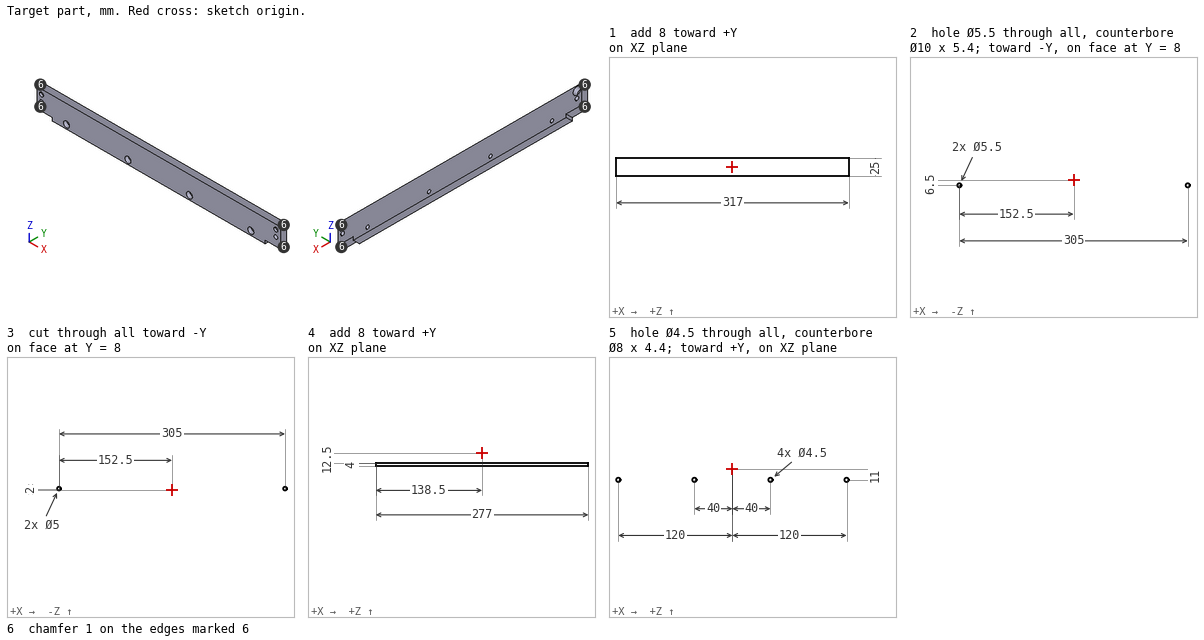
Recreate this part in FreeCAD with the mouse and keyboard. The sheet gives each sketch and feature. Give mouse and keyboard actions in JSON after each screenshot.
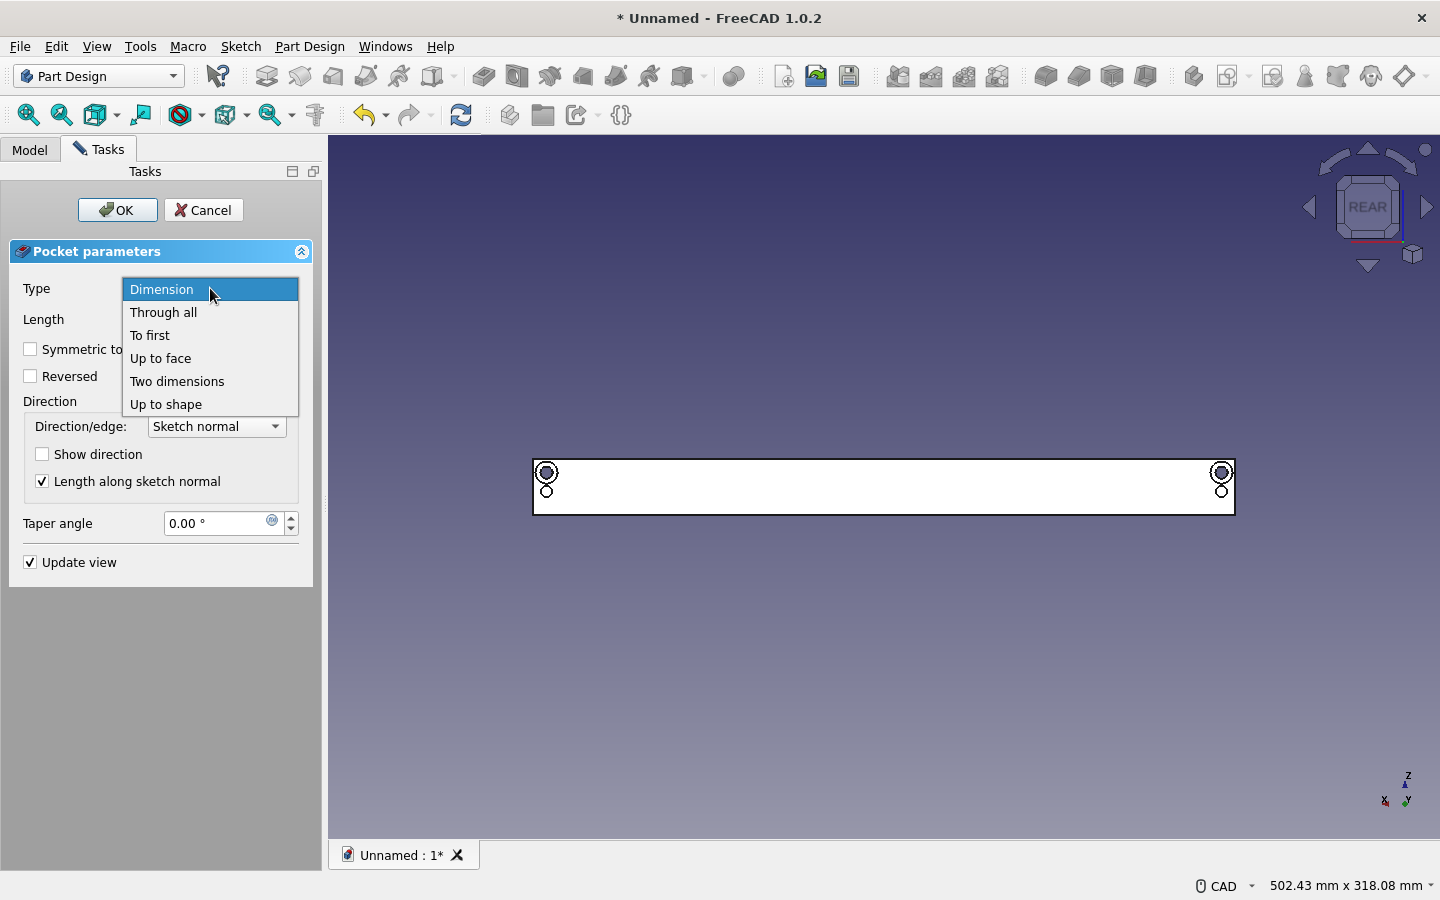
{"action": "left_click", "coordinate": [208, 312]}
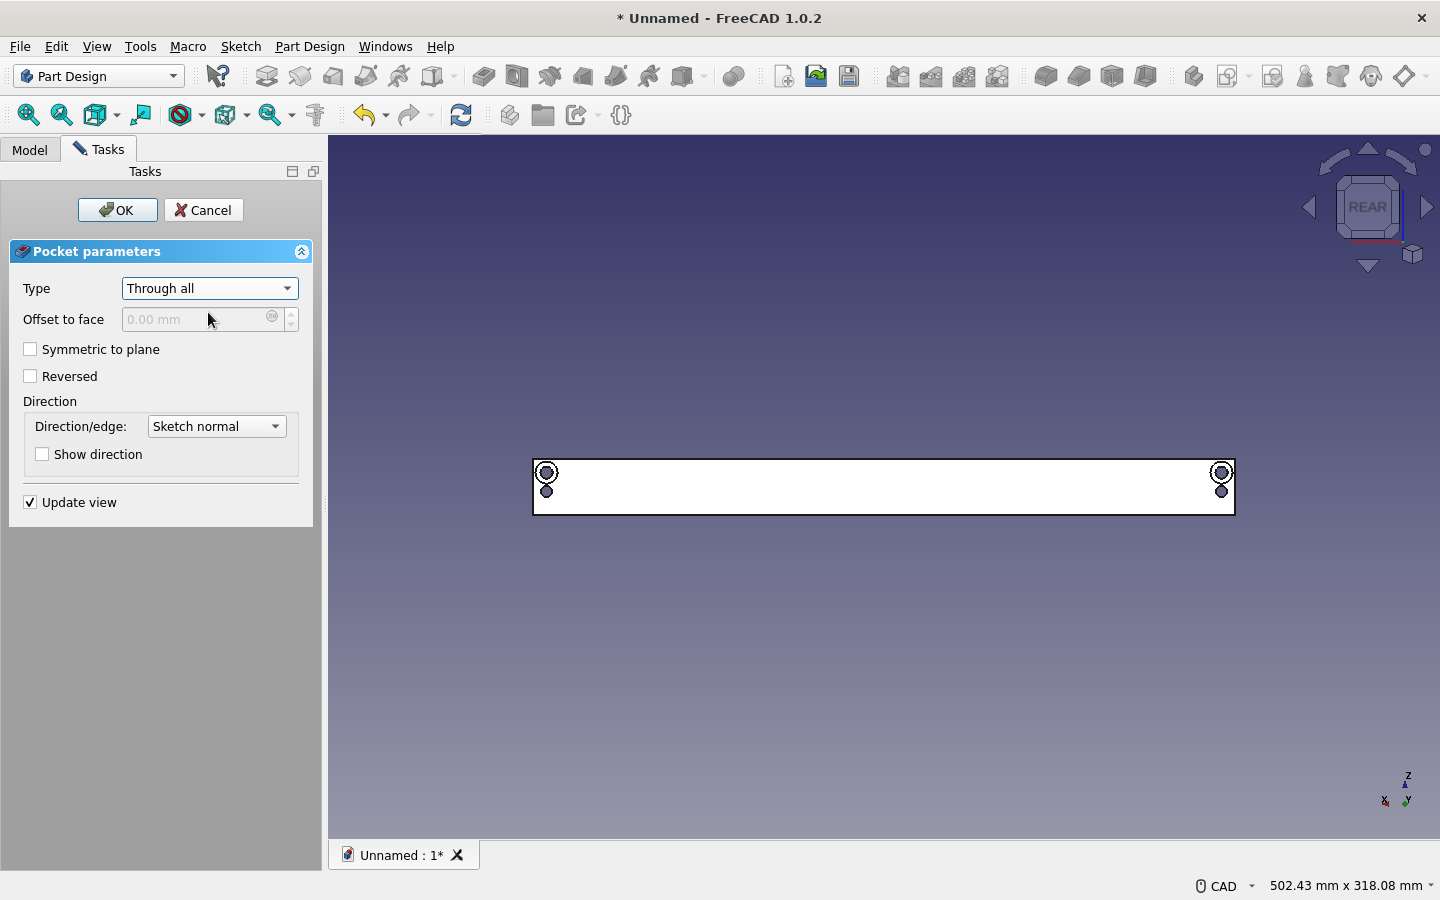
{"action": "left_click", "coordinate": [118, 210]}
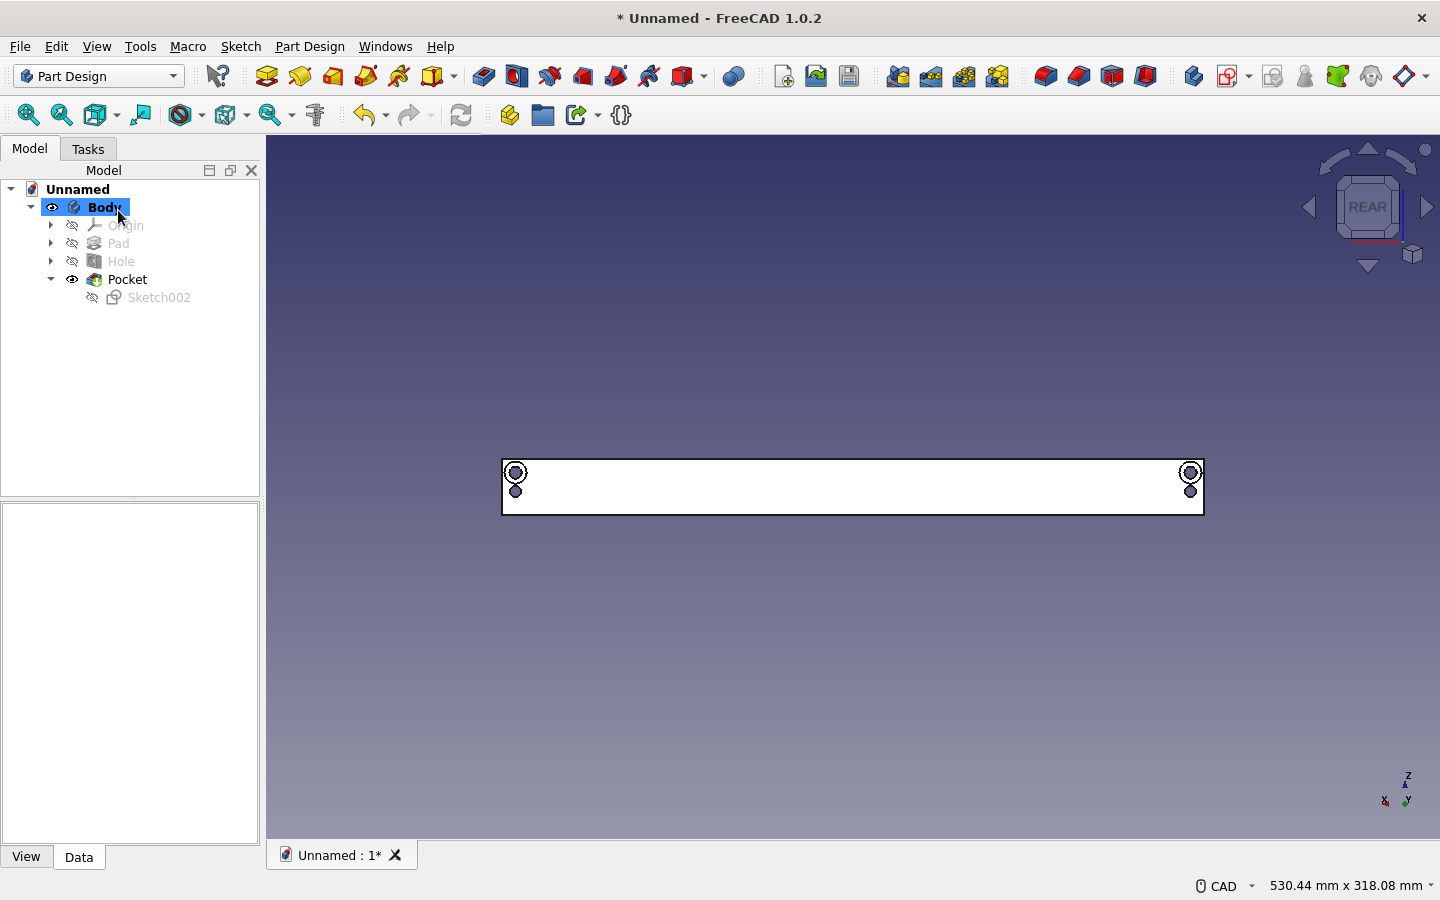
{"action": "left_click", "coordinate": [1226, 76]}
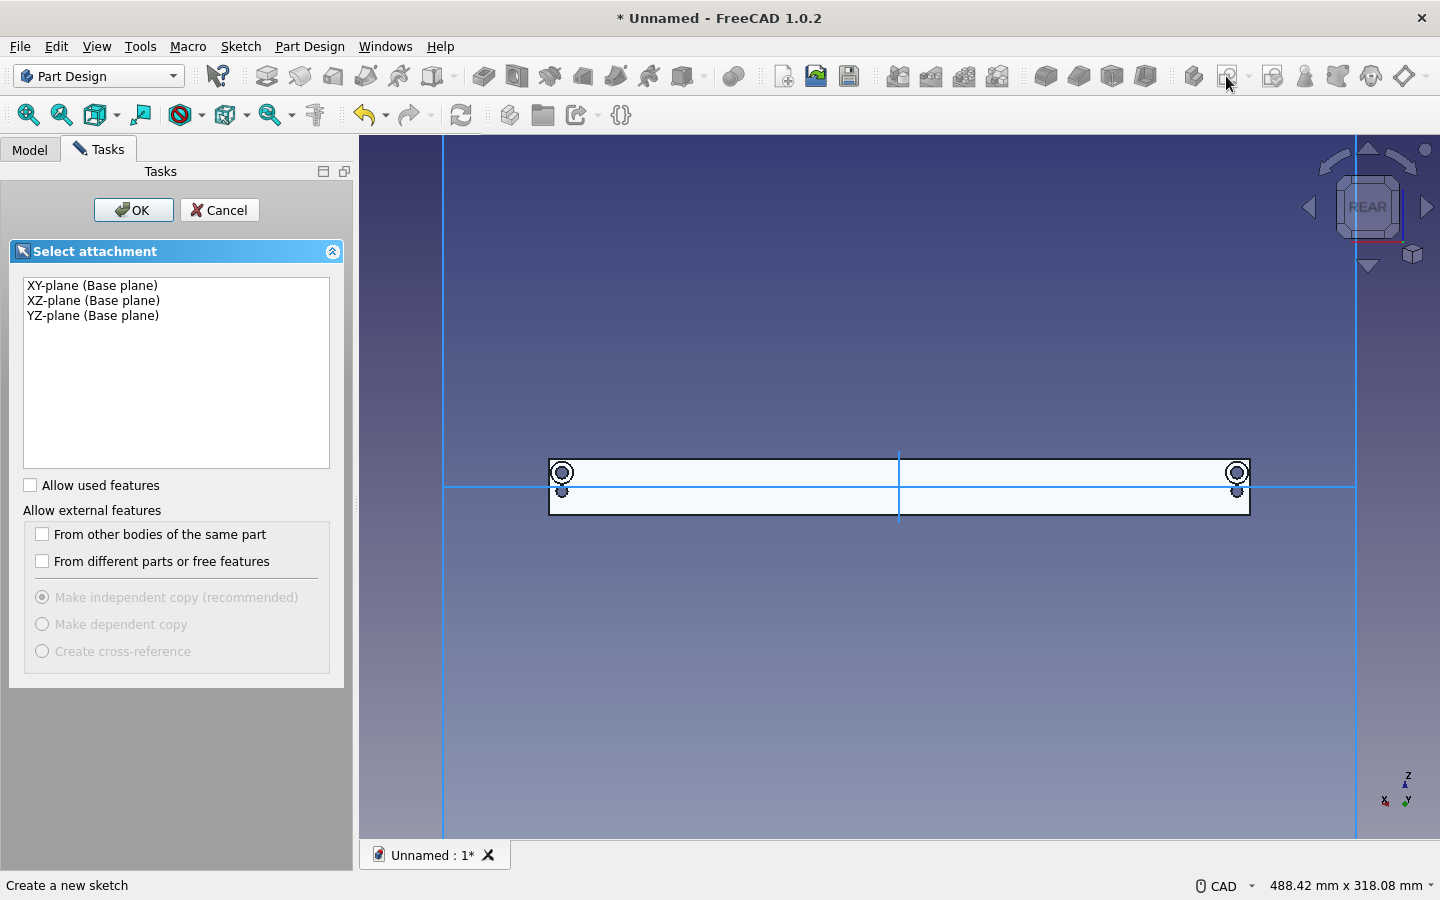
{"action": "left_click", "coordinate": [84, 300]}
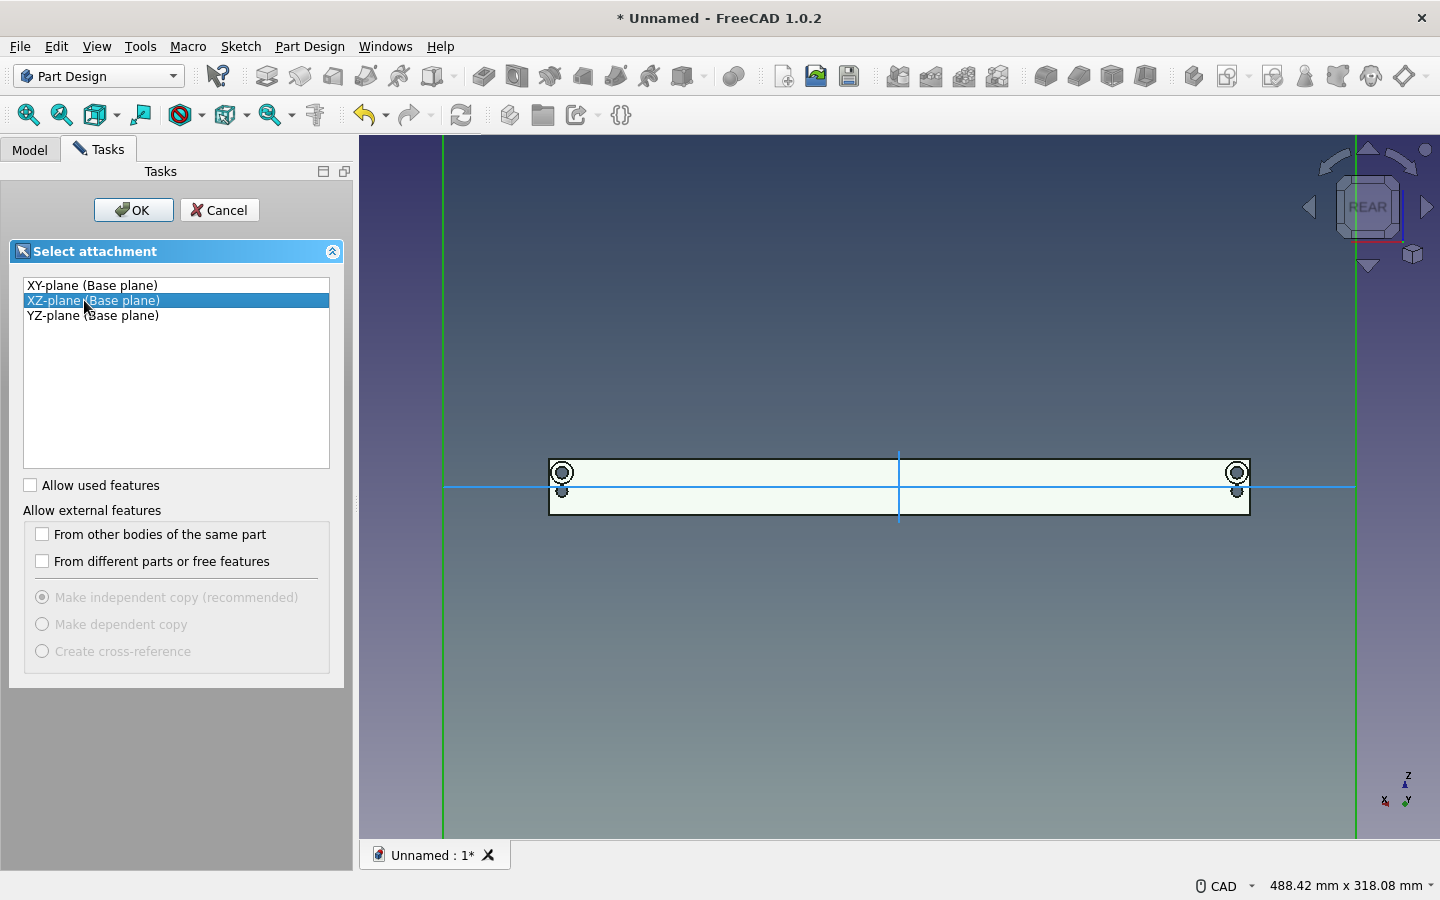
{"action": "left_click", "coordinate": [134, 210]}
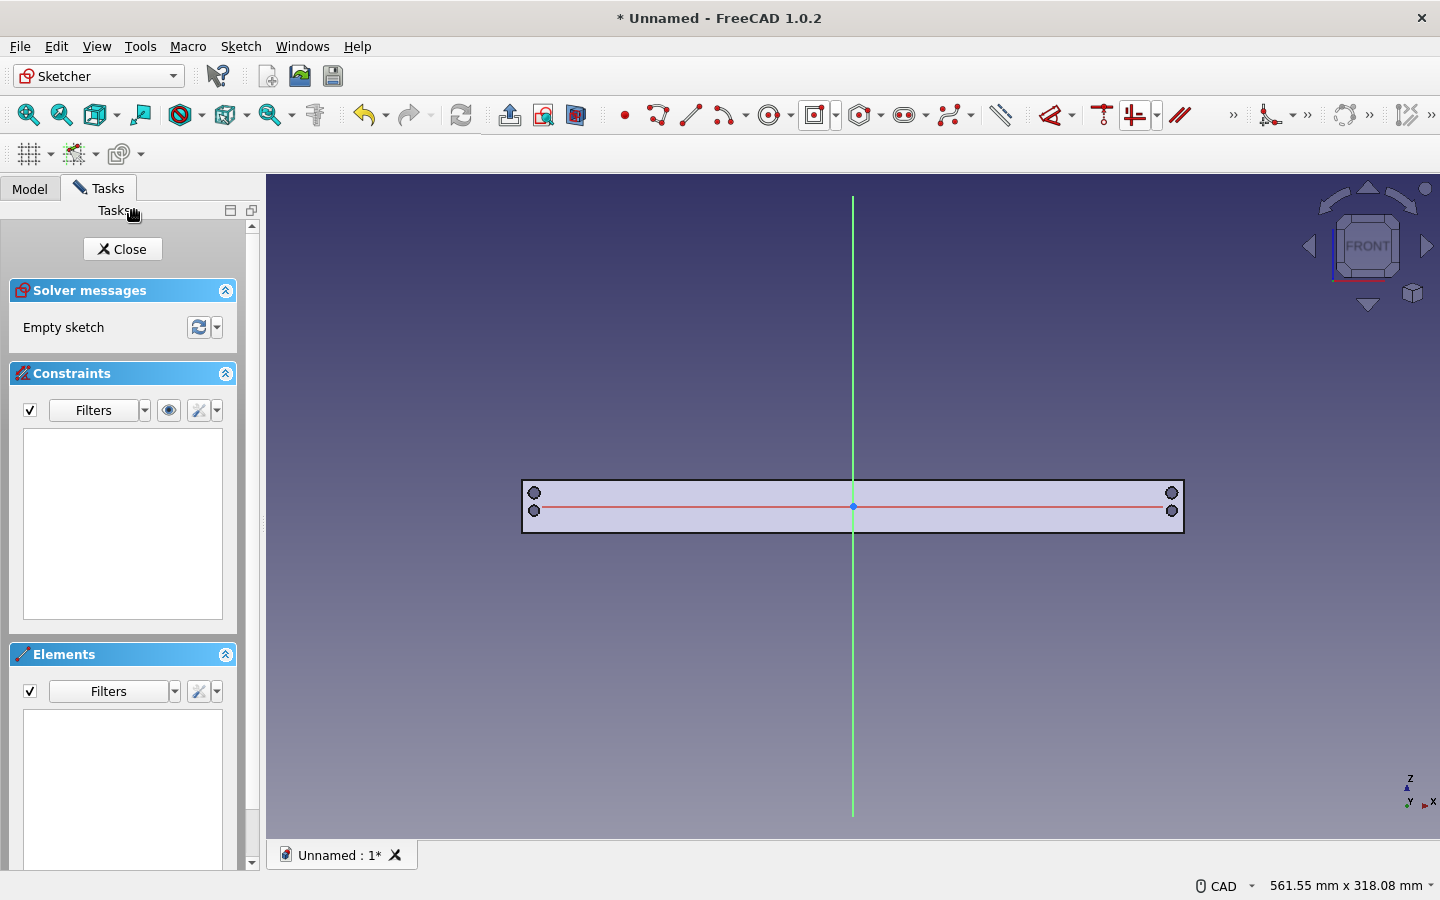
{"action": "left_click", "coordinate": [836, 116]}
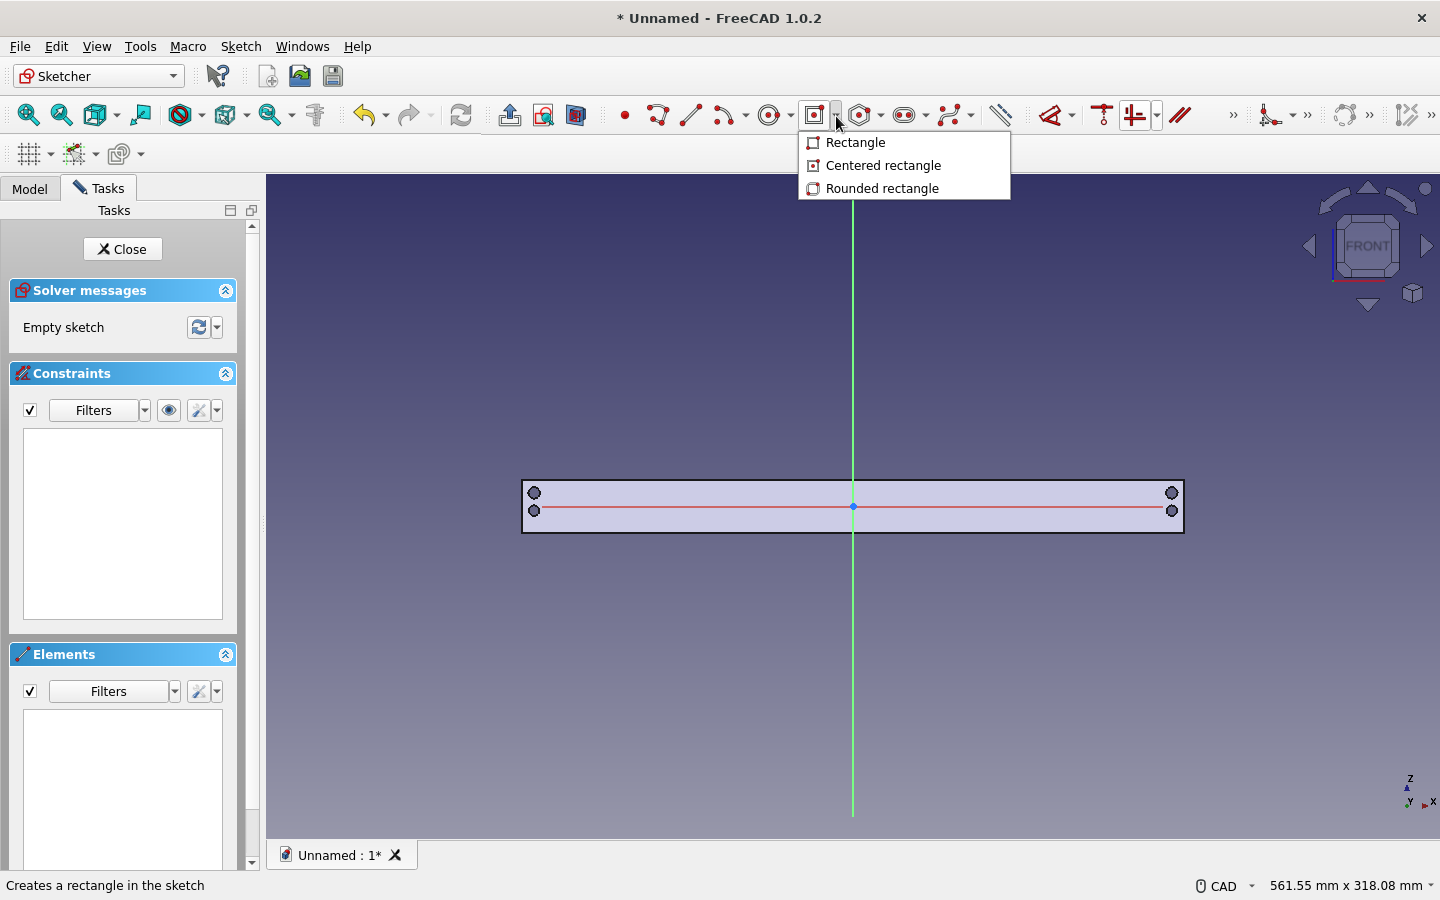
{"action": "left_click", "coordinate": [904, 142]}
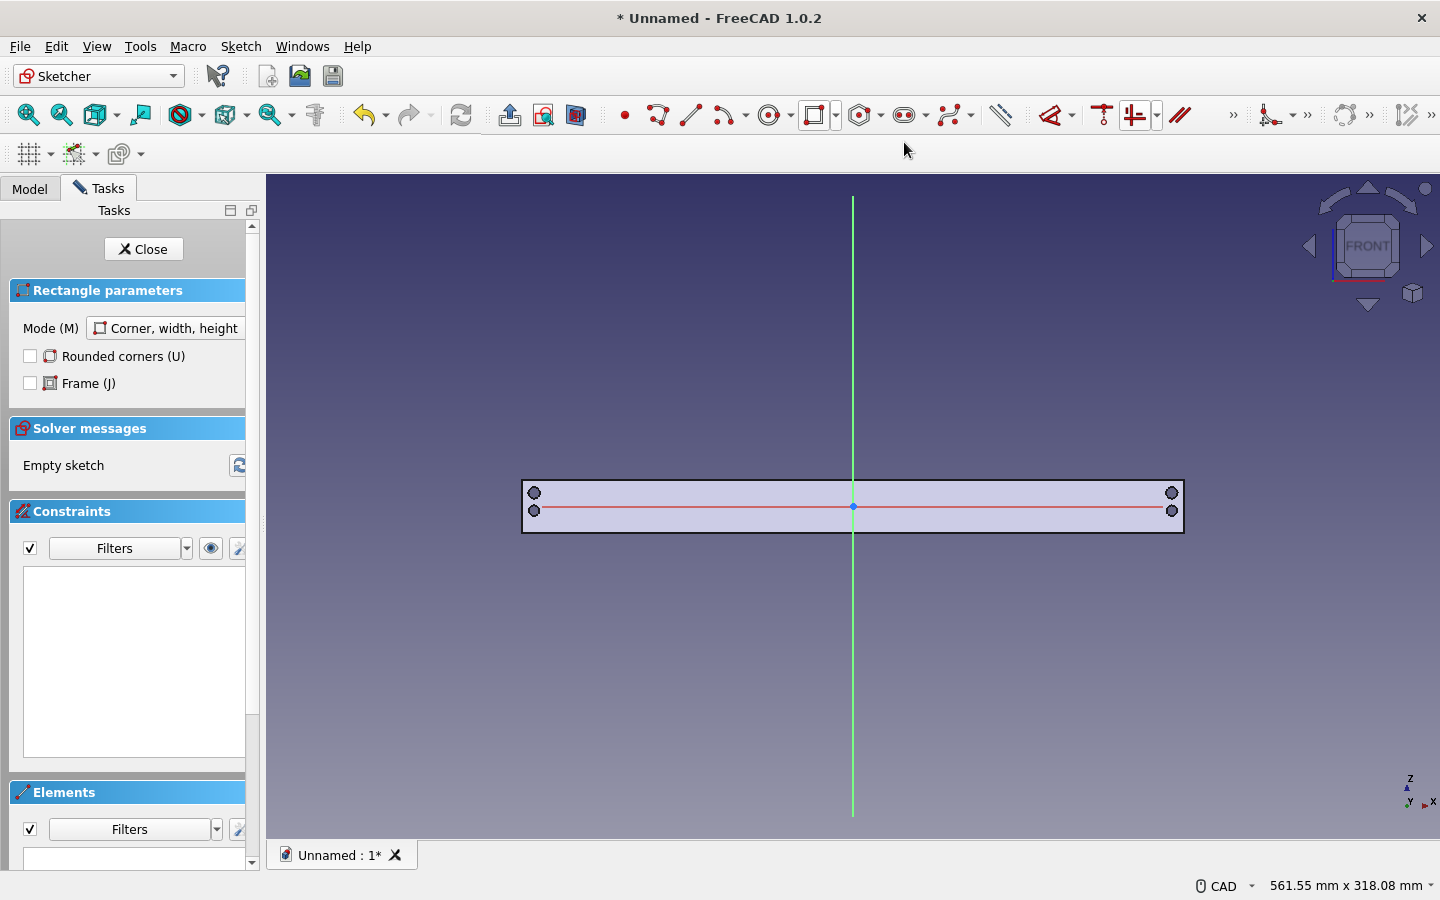
{"action": "scroll", "coordinate": [563, 533], "scroll_direction": "up", "scroll_amount": 4}